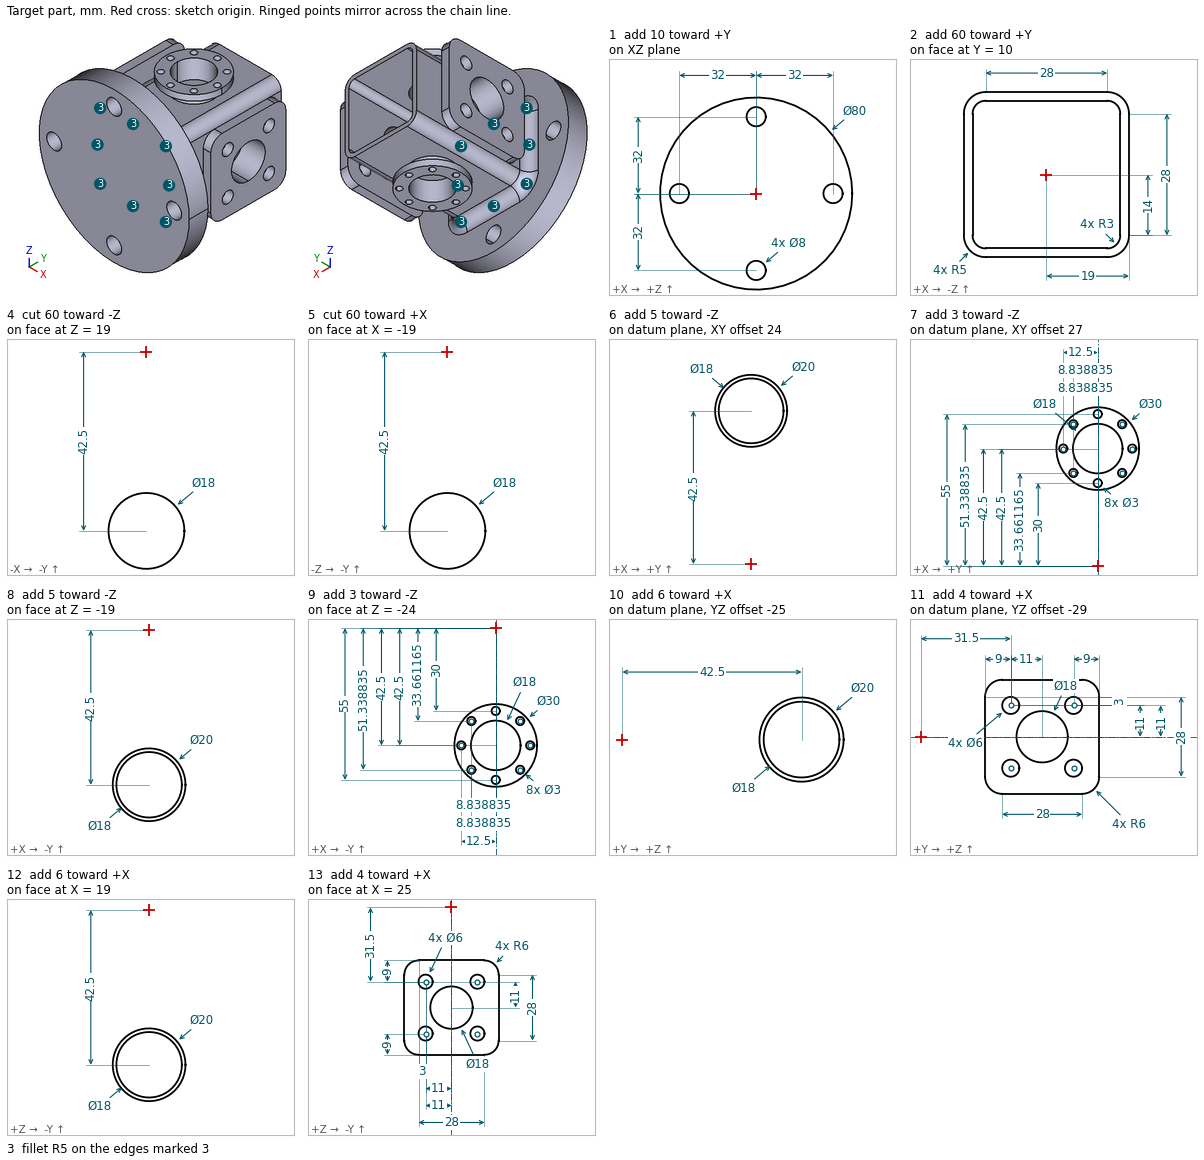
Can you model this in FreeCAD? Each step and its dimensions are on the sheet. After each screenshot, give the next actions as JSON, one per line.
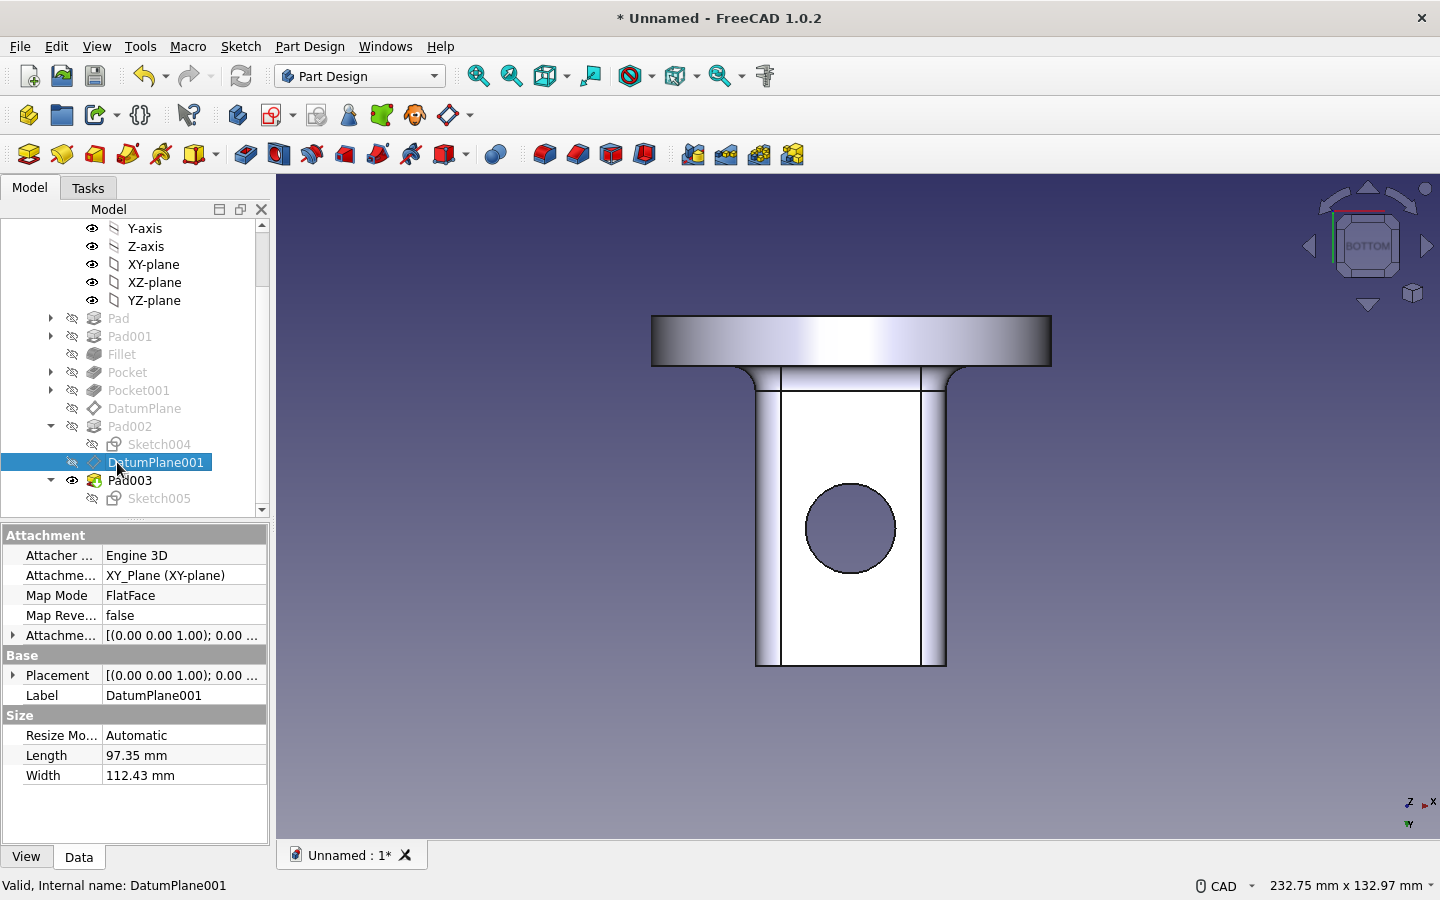
{"action": "left_click", "coordinate": [831, 606]}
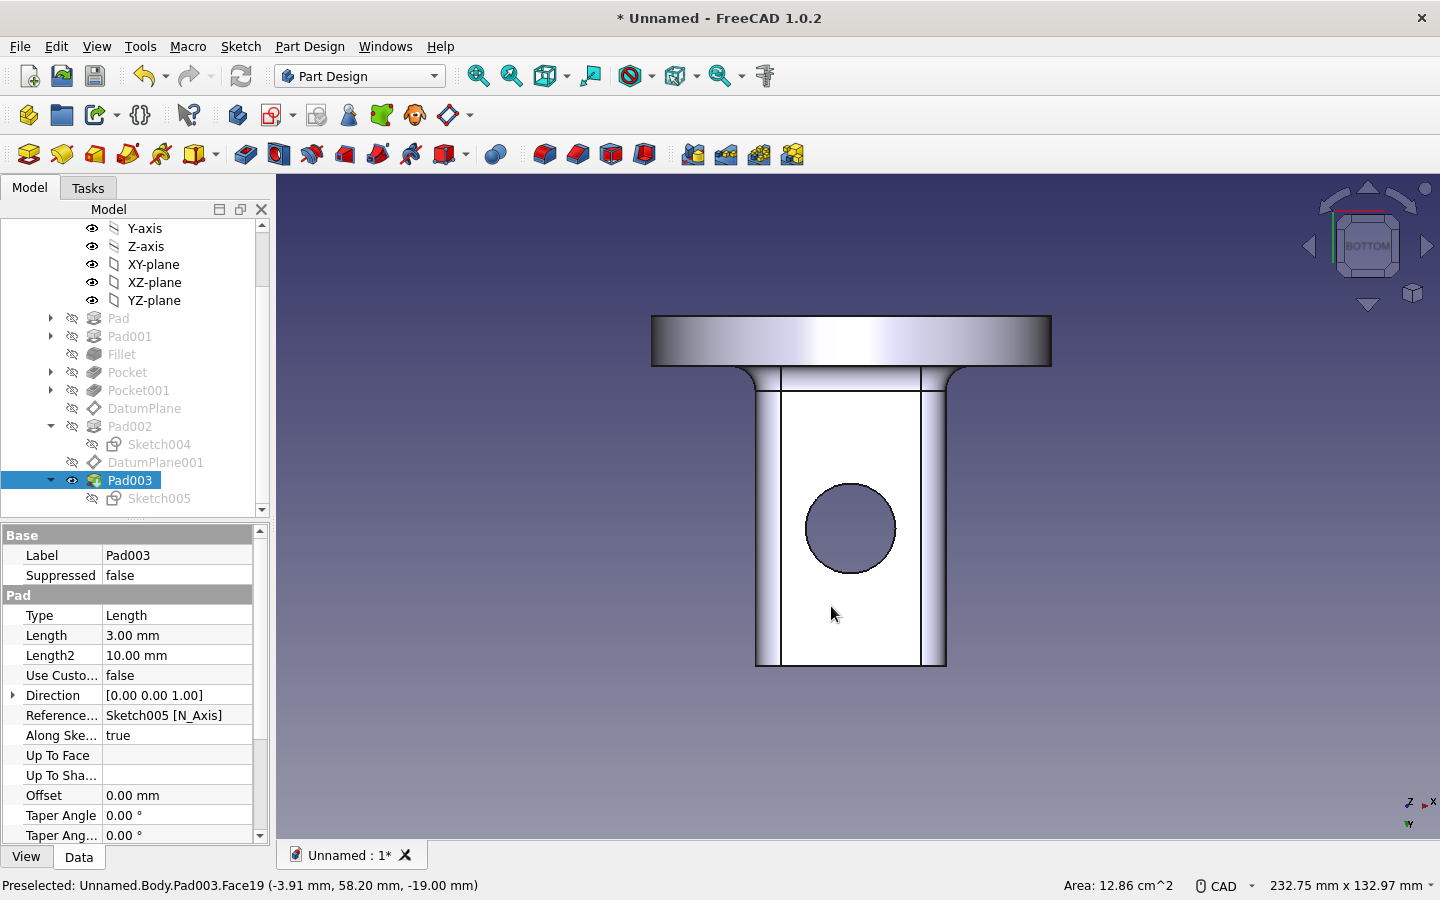
{"action": "left_click", "coordinate": [270, 116]}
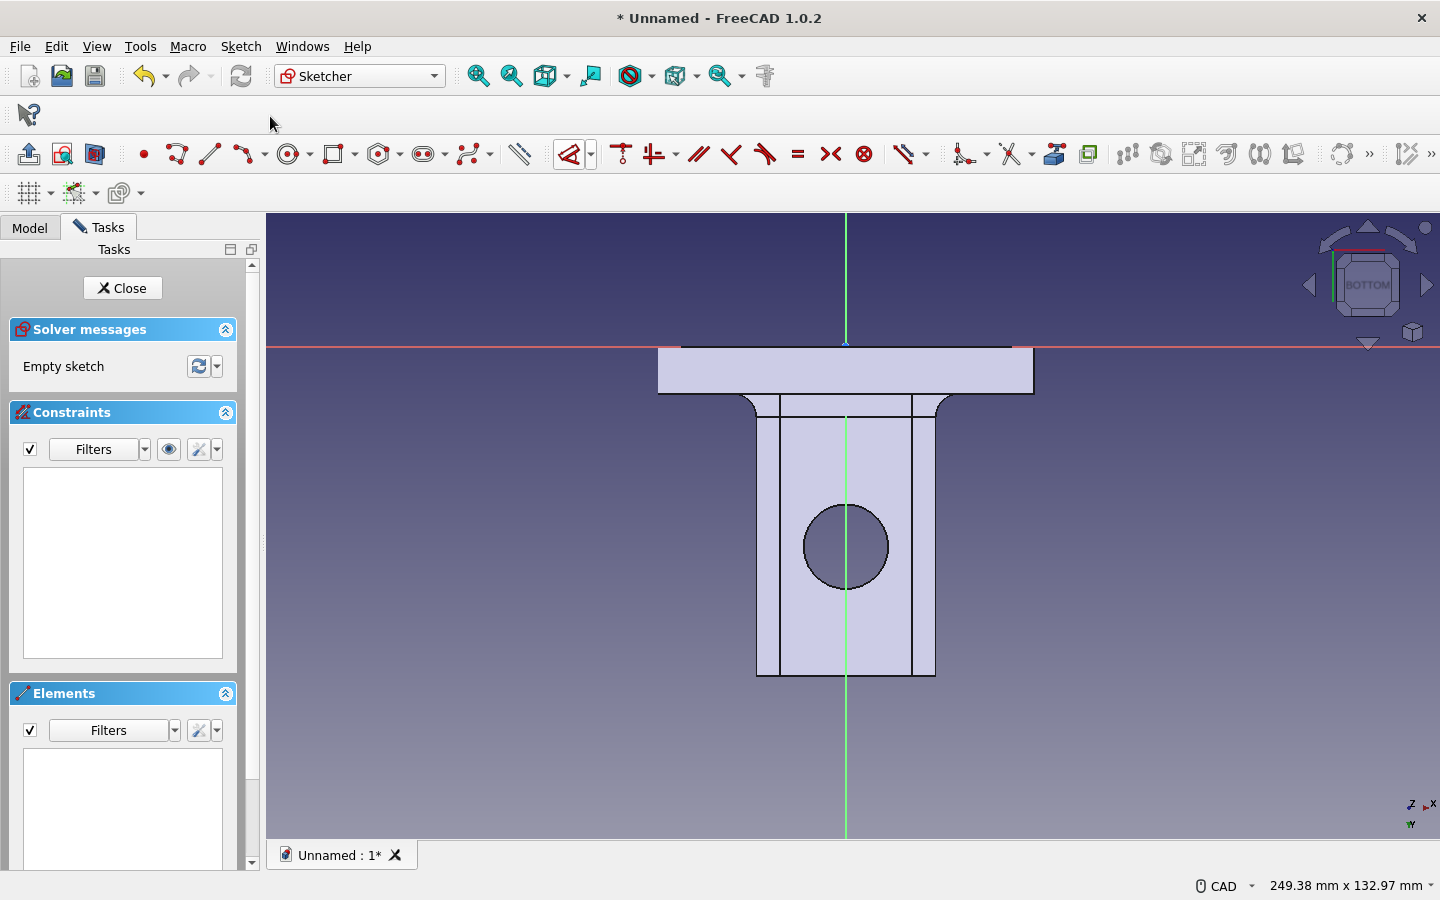
{"action": "scroll", "coordinate": [866, 553], "scroll_direction": "up", "scroll_amount": 7}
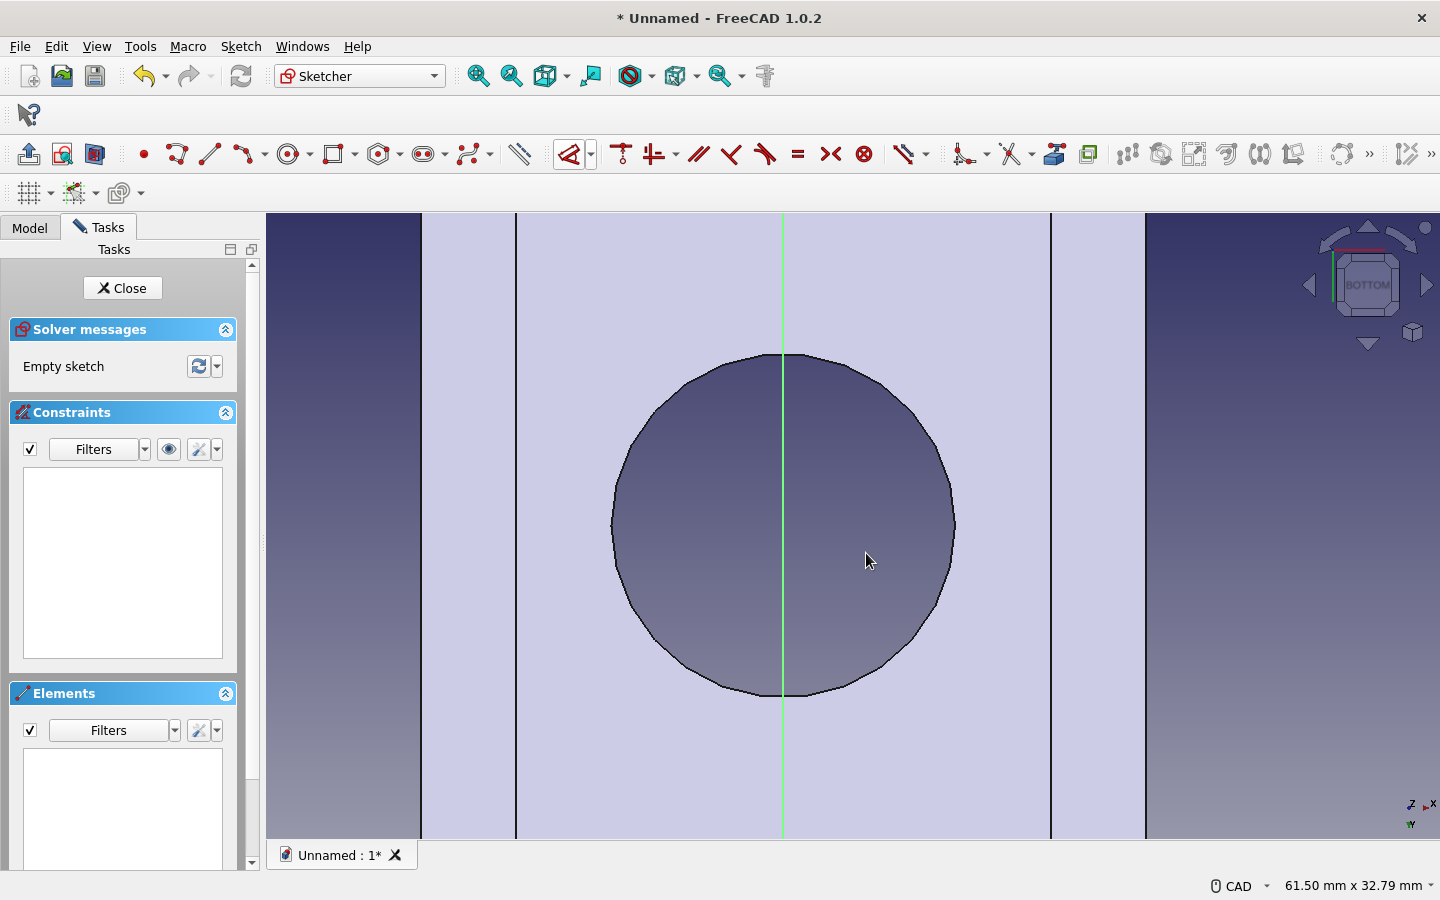
{"action": "key", "text": "g c"}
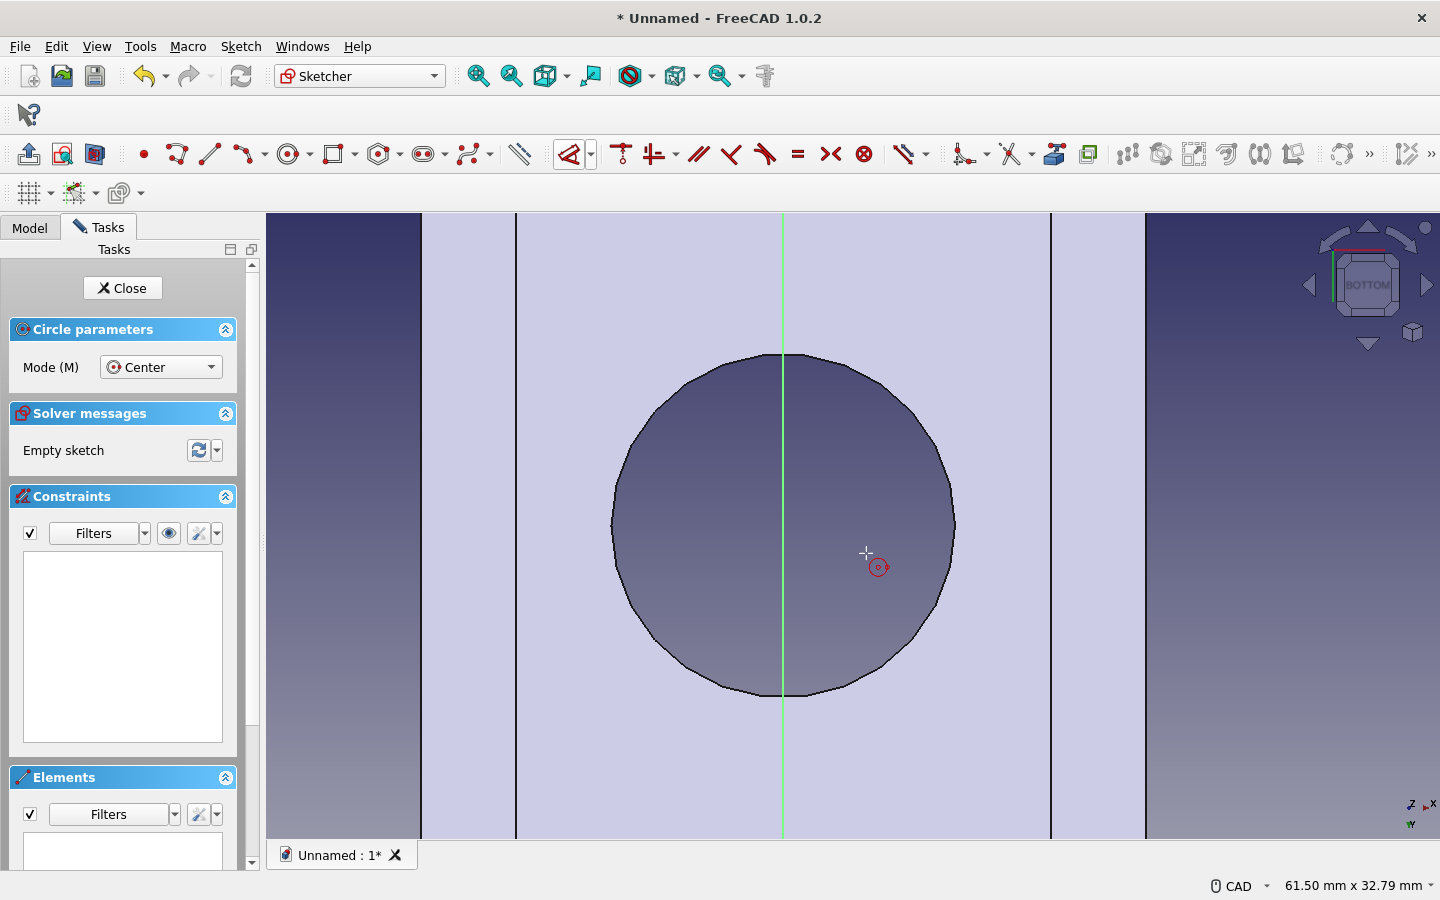
{"action": "left_click", "coordinate": [783, 526]}
{"action": "mouse_move", "coordinate": [918, 391]}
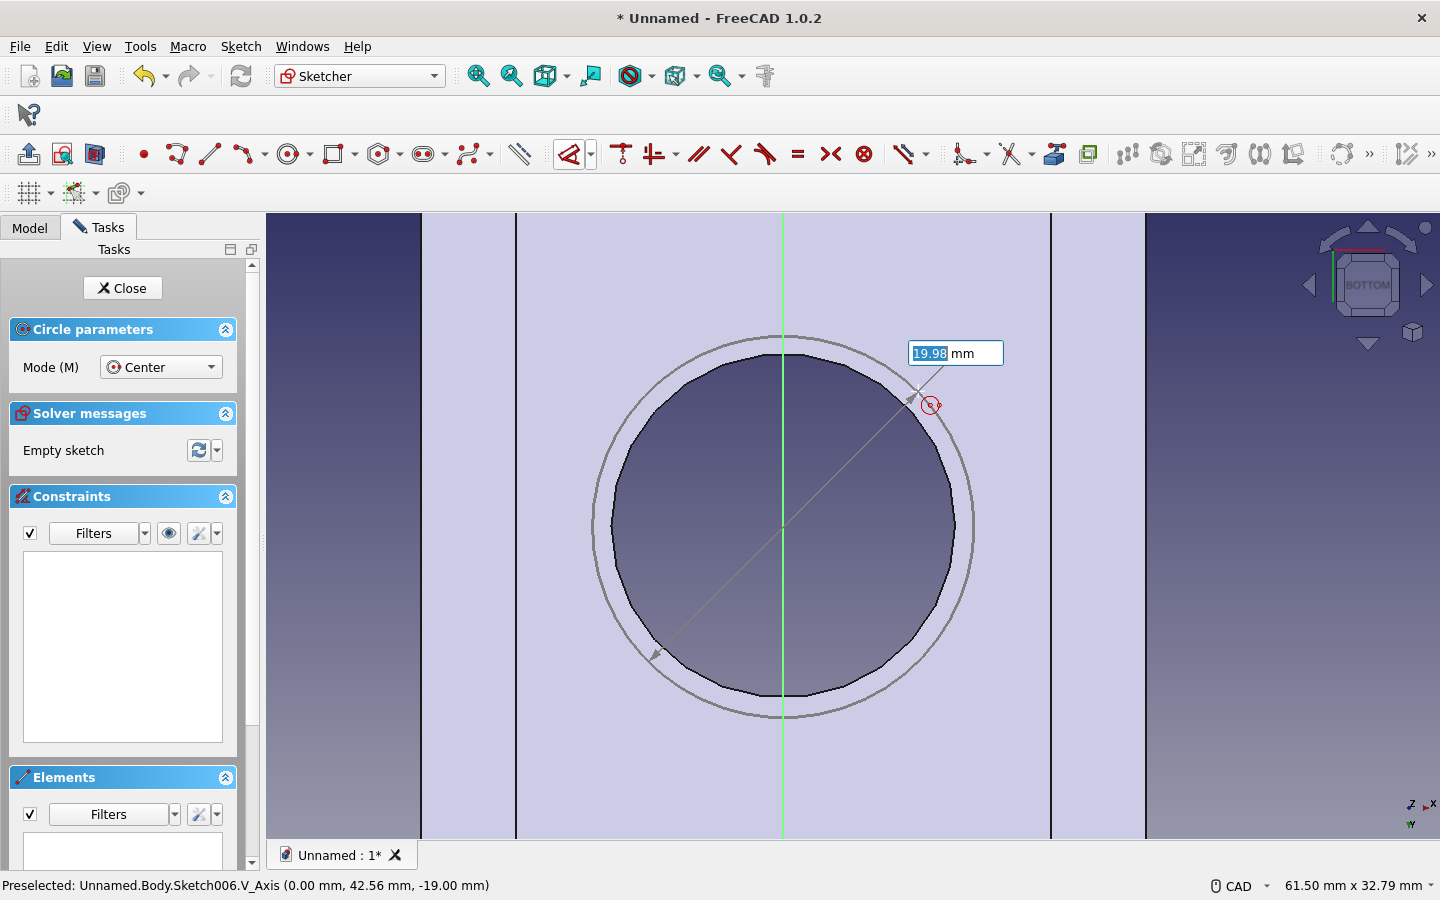
{"action": "type", "text": "20"}
{"action": "key", "text": "Return"}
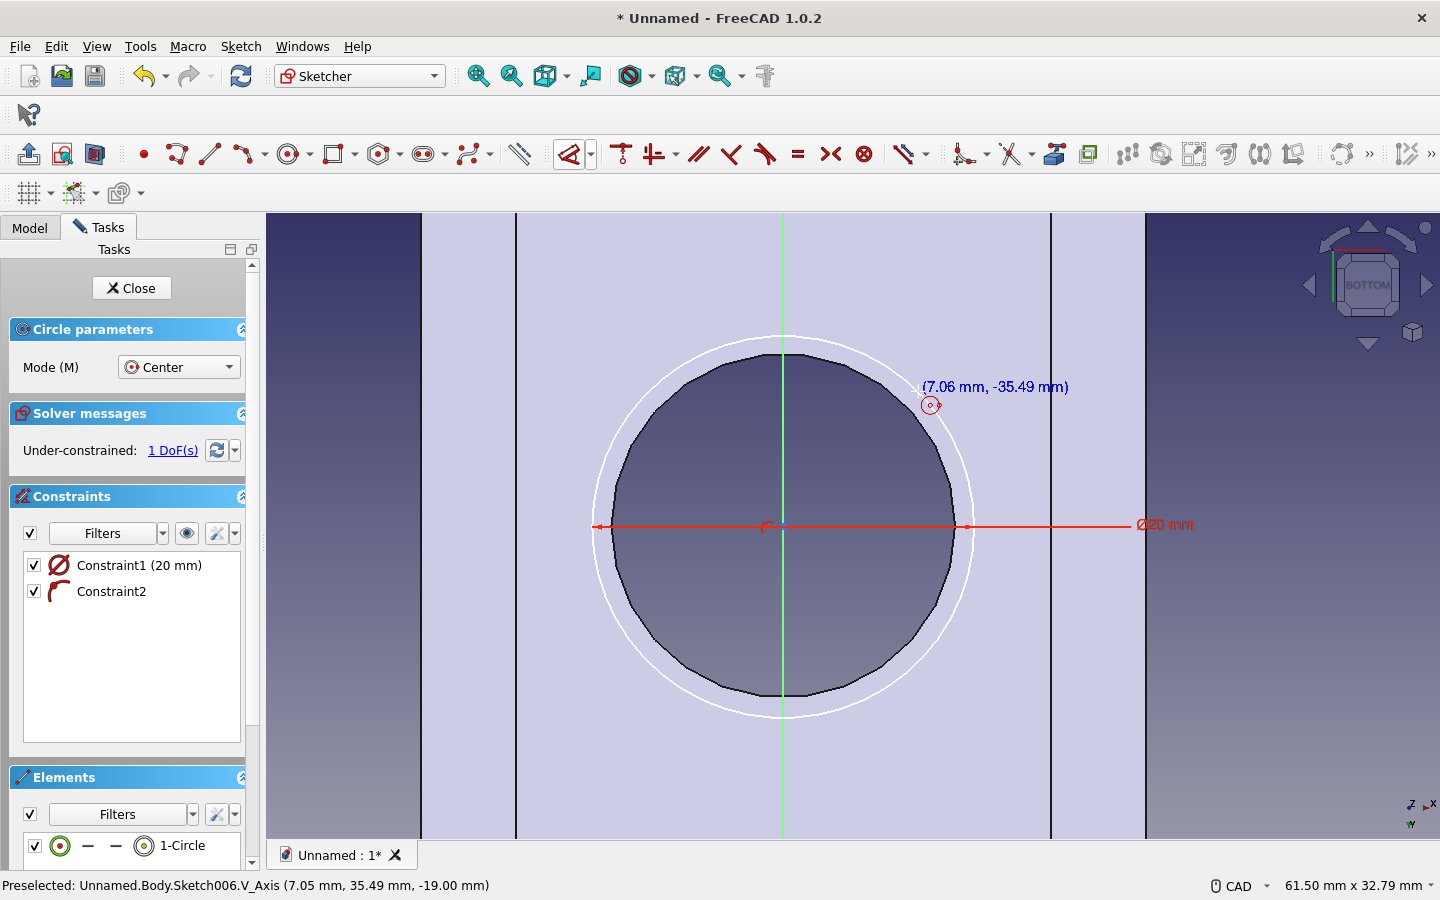
{"action": "left_click", "coordinate": [783, 527]}
{"action": "mouse_move", "coordinate": [905, 404]}